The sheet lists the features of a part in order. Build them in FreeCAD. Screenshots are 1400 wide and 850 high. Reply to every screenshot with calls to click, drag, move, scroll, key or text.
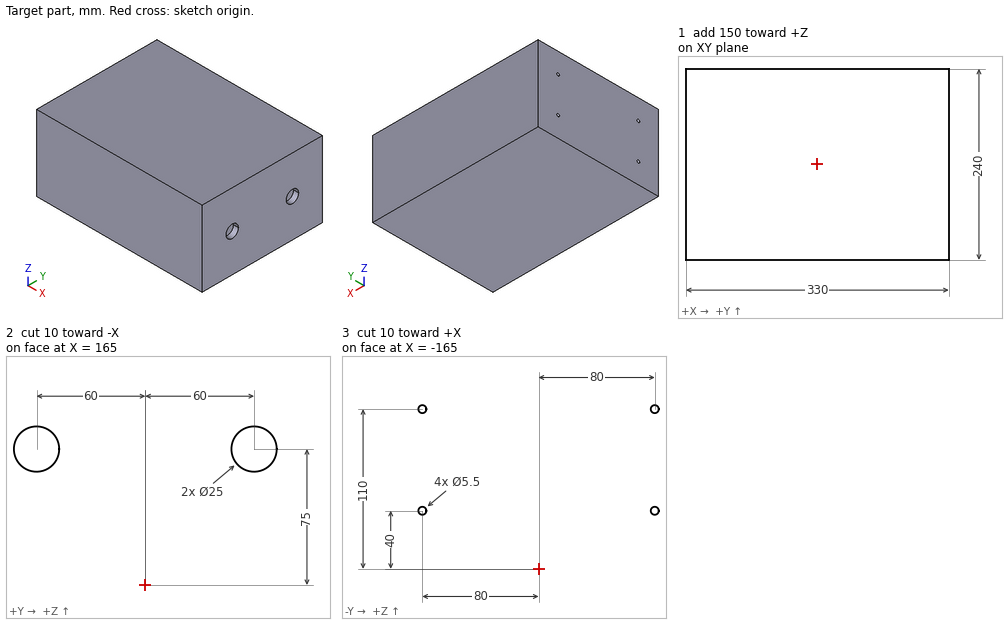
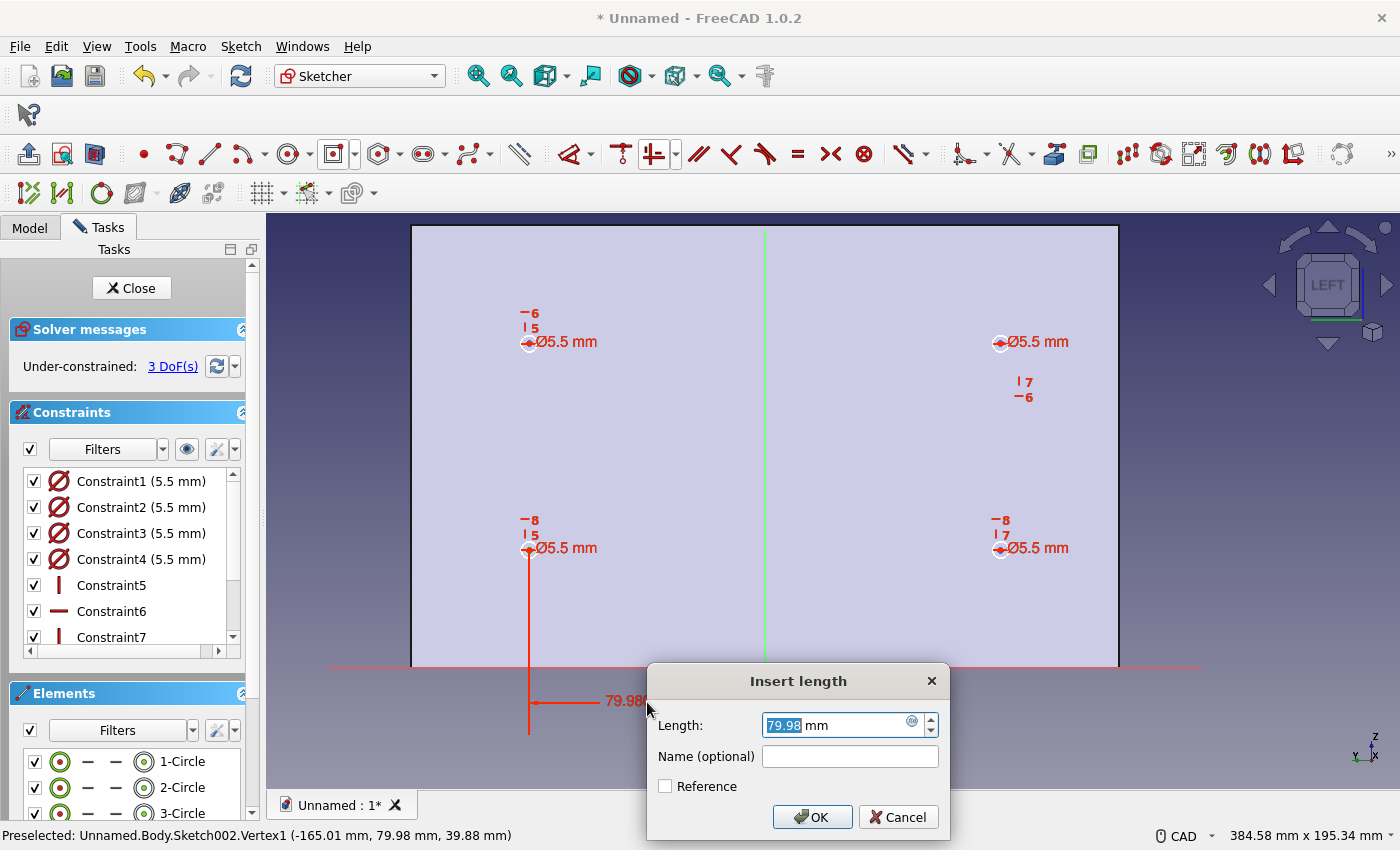
text(80)
key(Return)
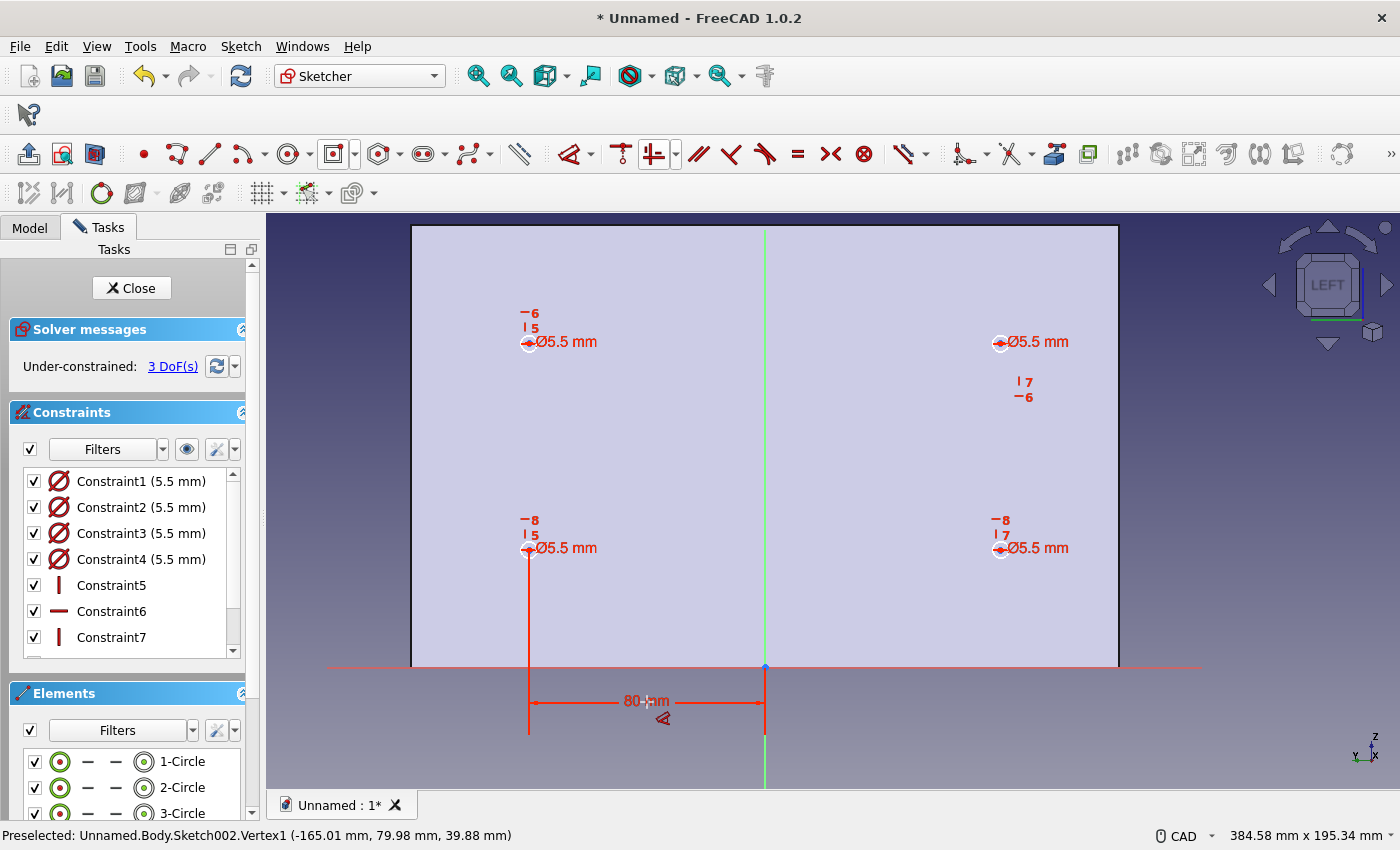
click(529, 550)
click(495, 609)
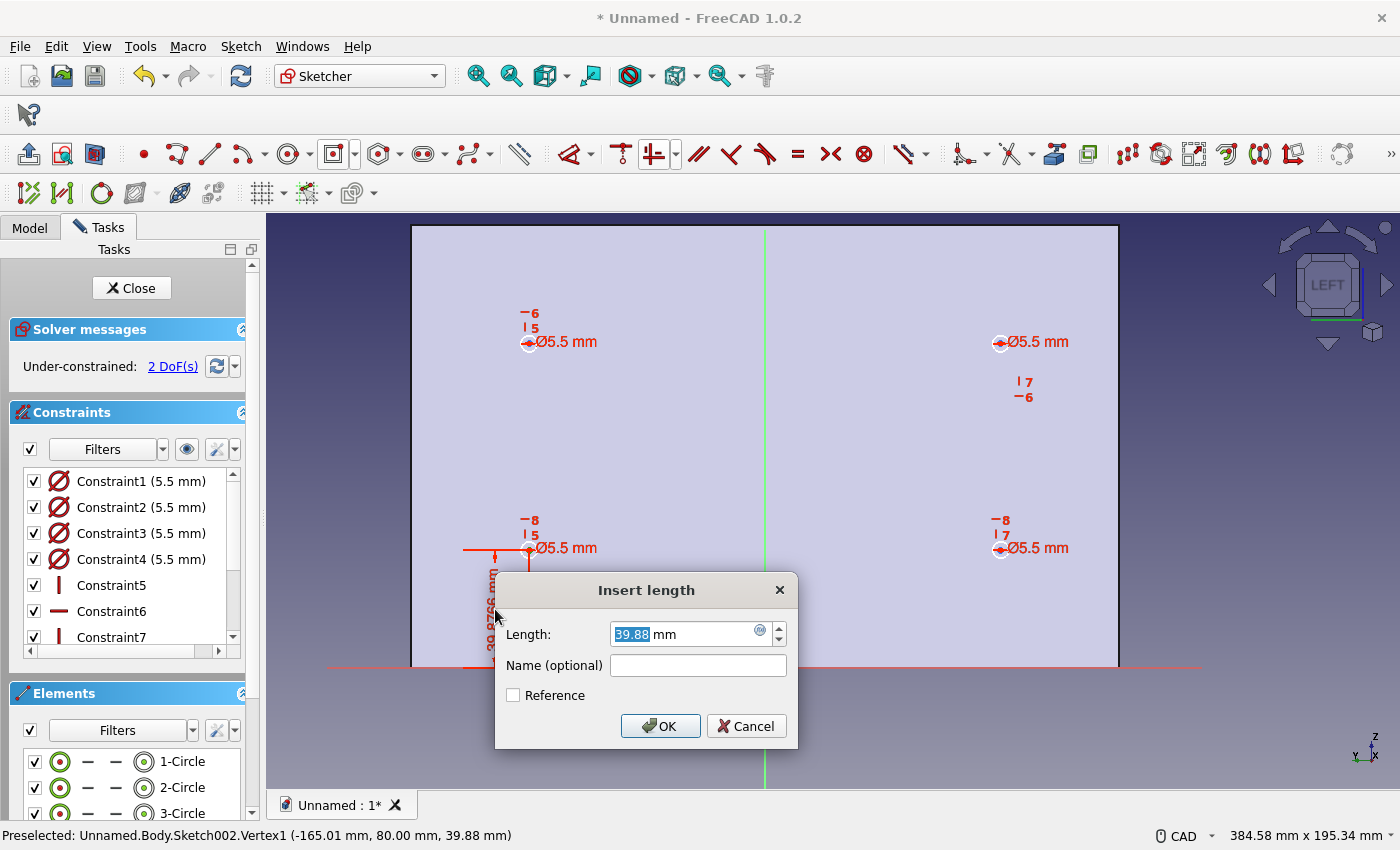
text(40)
key(Return)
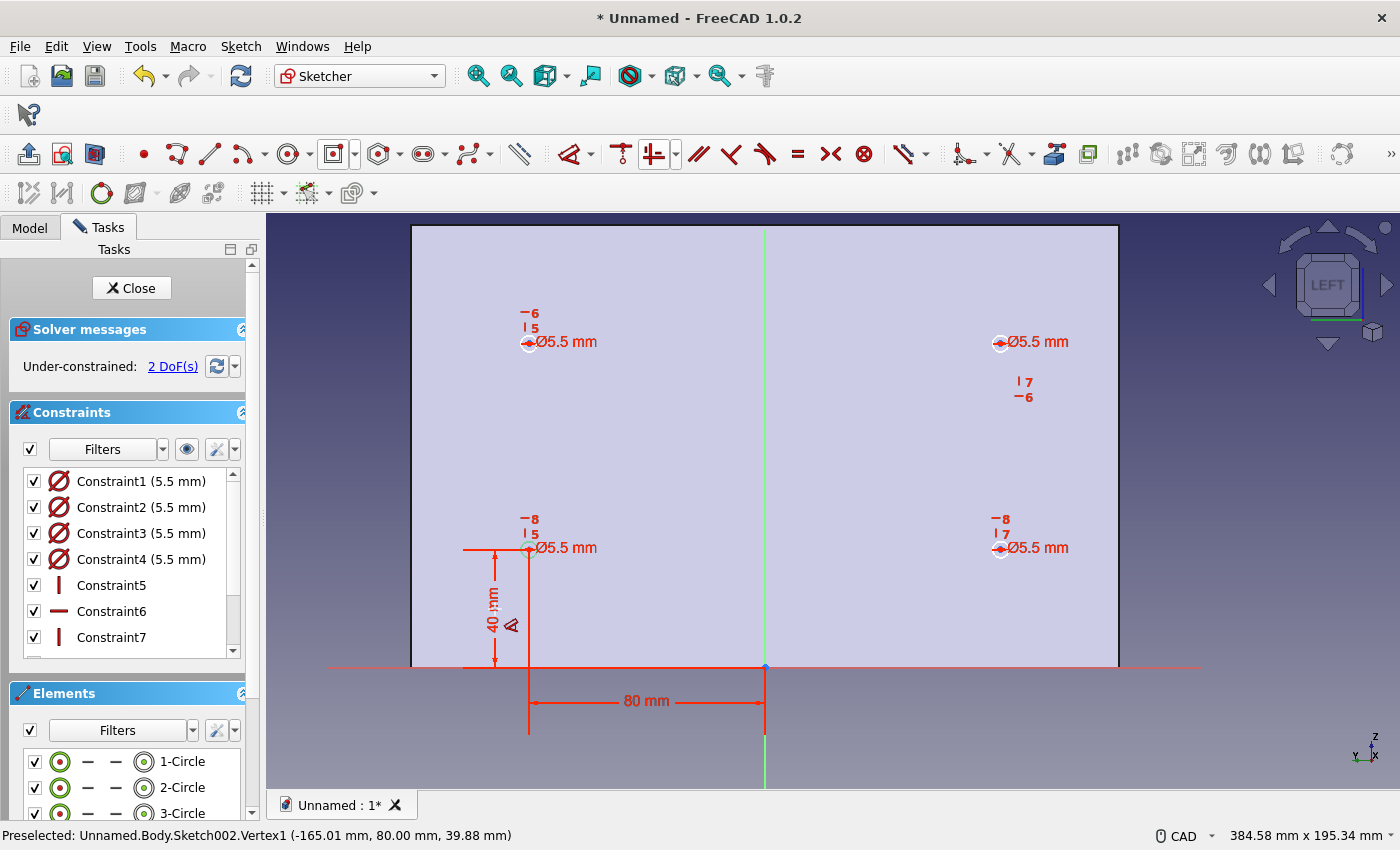
click(1001, 344)
click(883, 702)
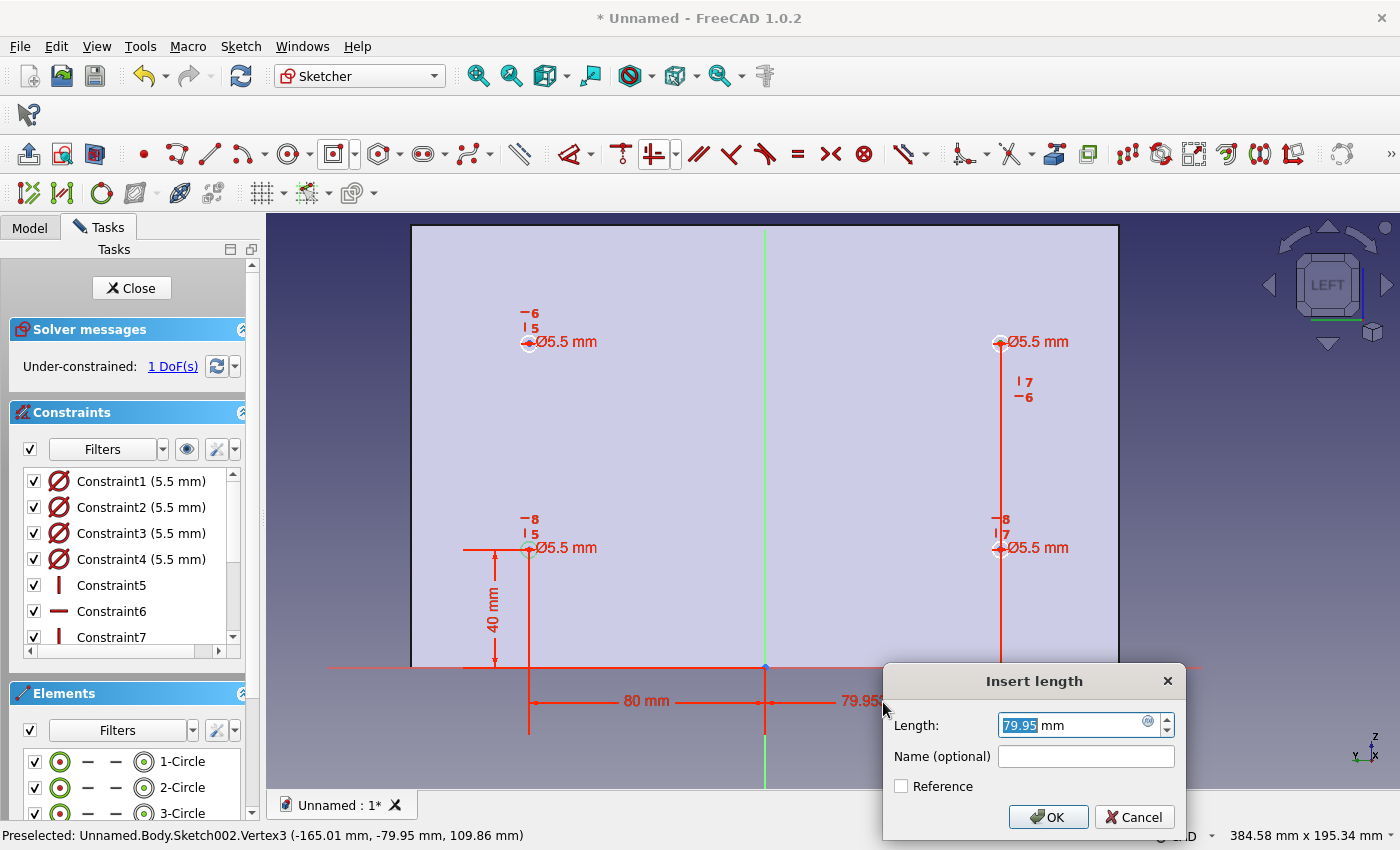
text(80)
key(Return)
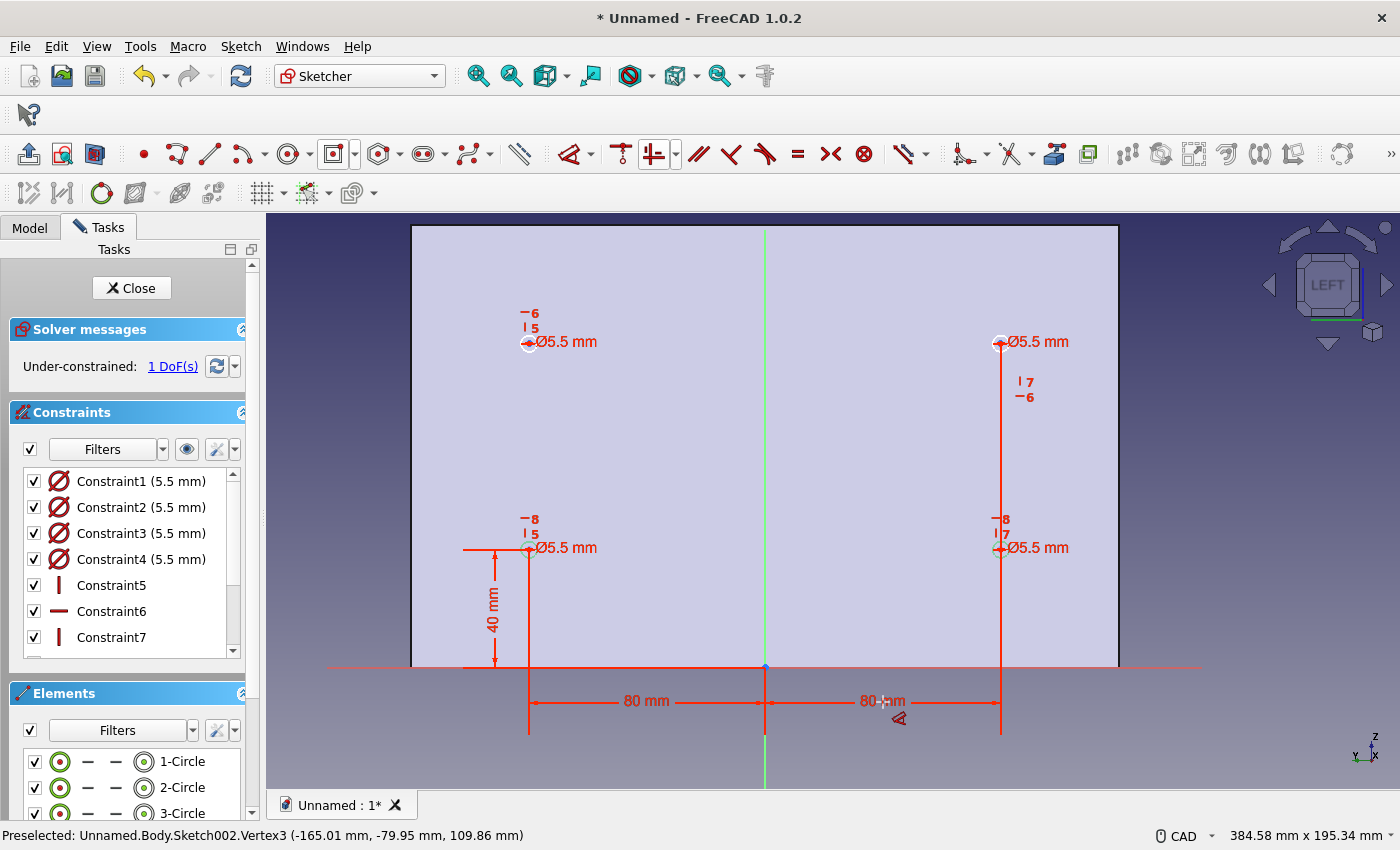
click(529, 344)
click(495, 506)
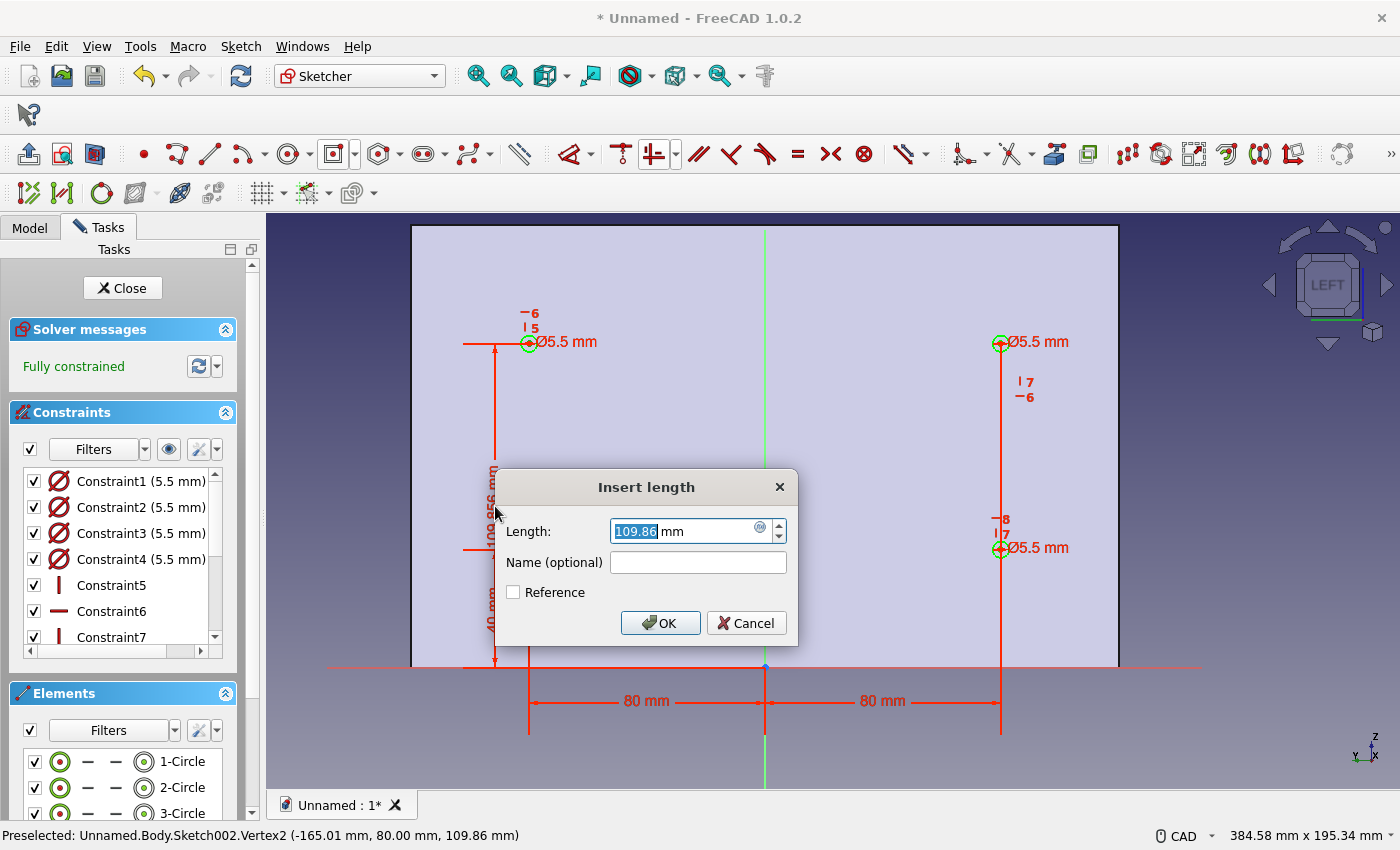
text(110)
key(Return)
key(Escape)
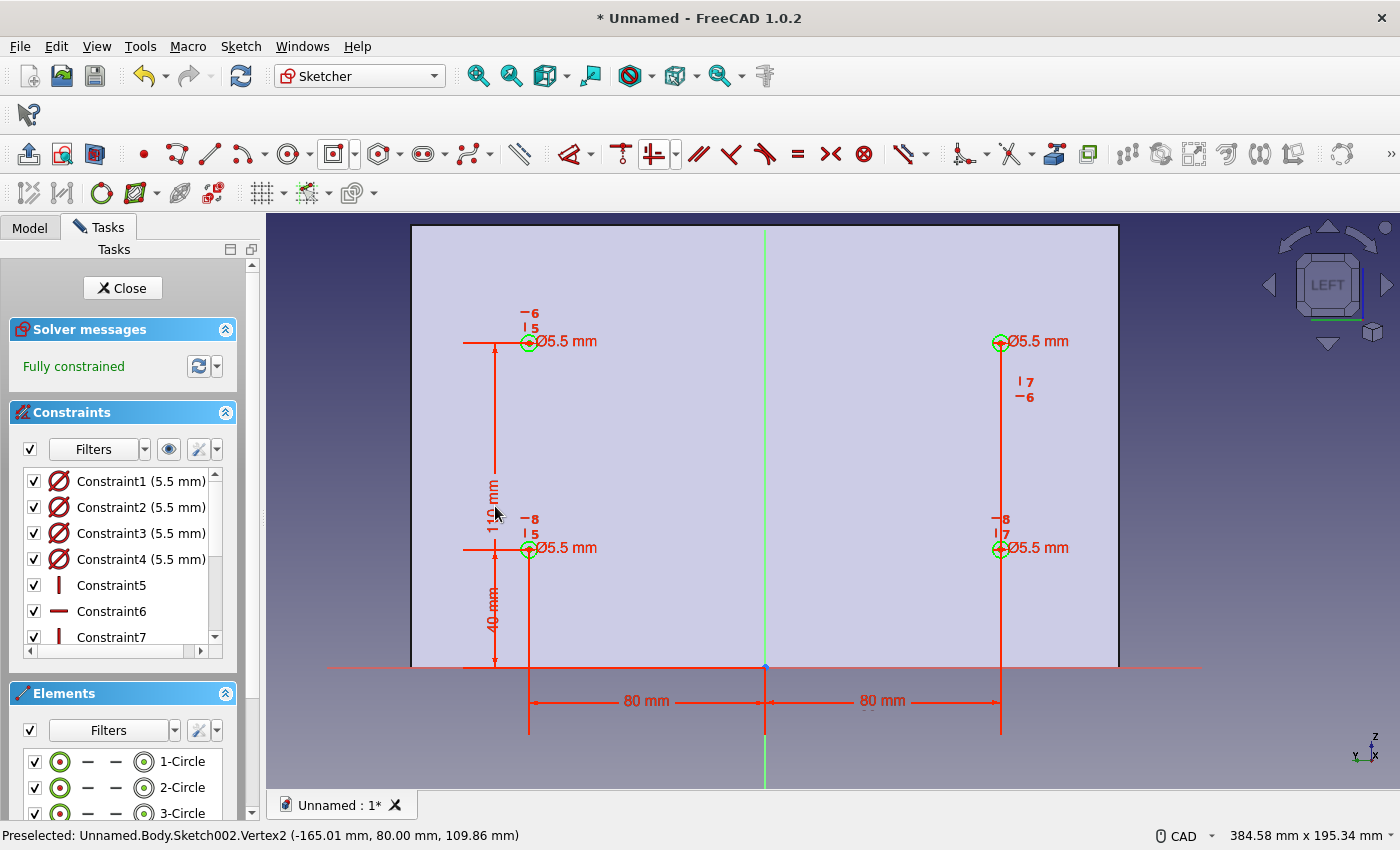
click(123, 288)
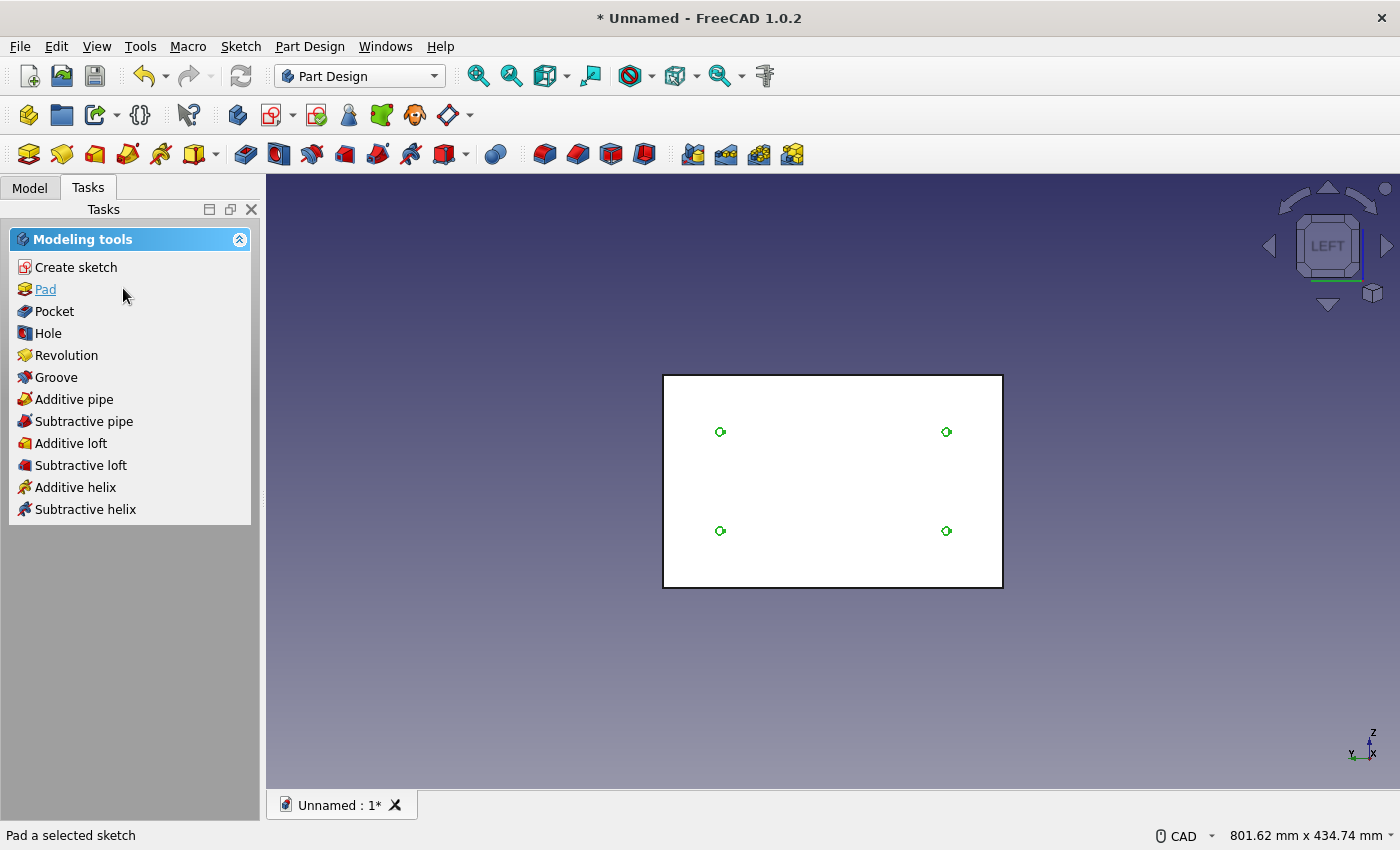
click(246, 154)